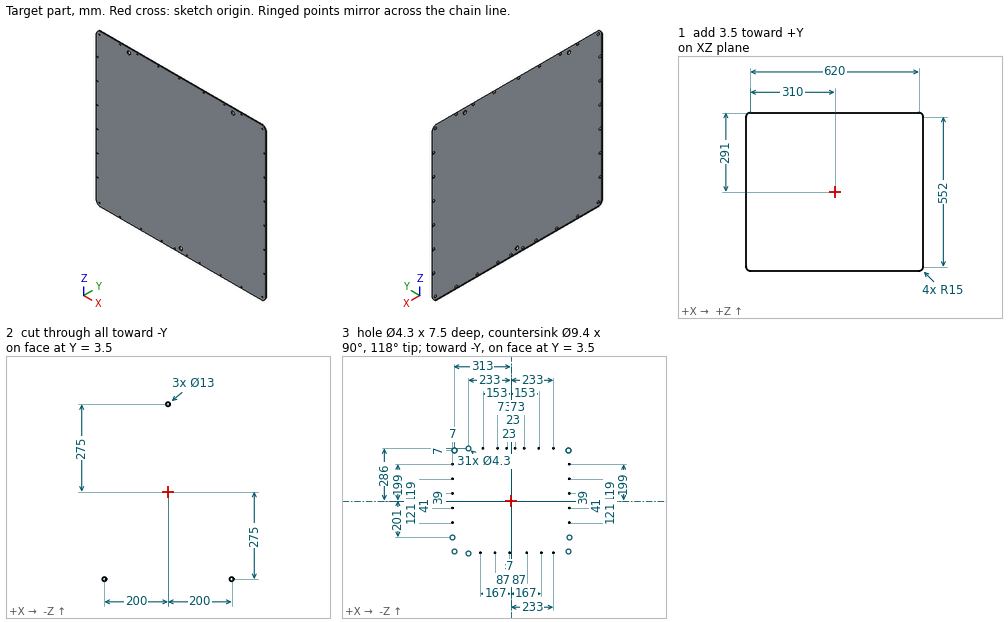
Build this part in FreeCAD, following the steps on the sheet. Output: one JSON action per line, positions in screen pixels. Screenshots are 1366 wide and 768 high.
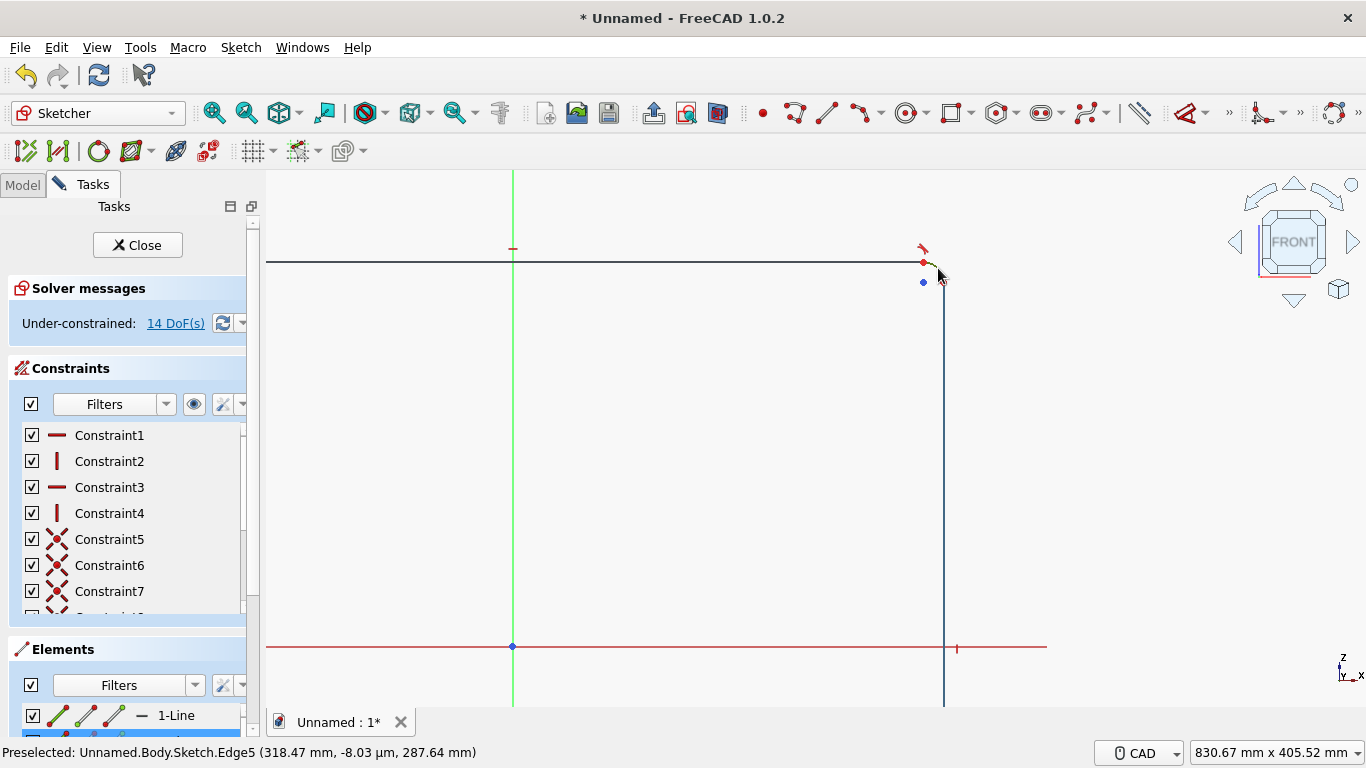
{"action": "key", "text": "t"}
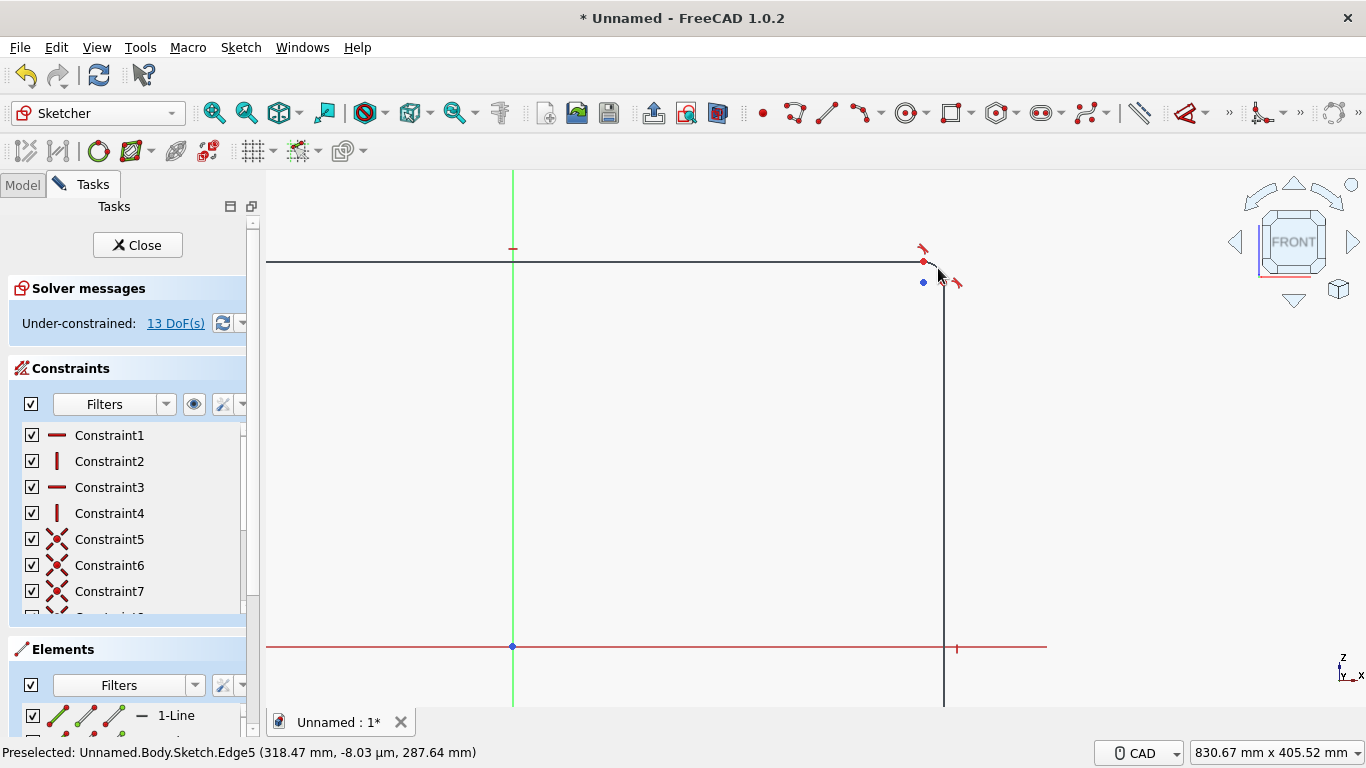
{"action": "left_click", "coordinate": [944, 502]}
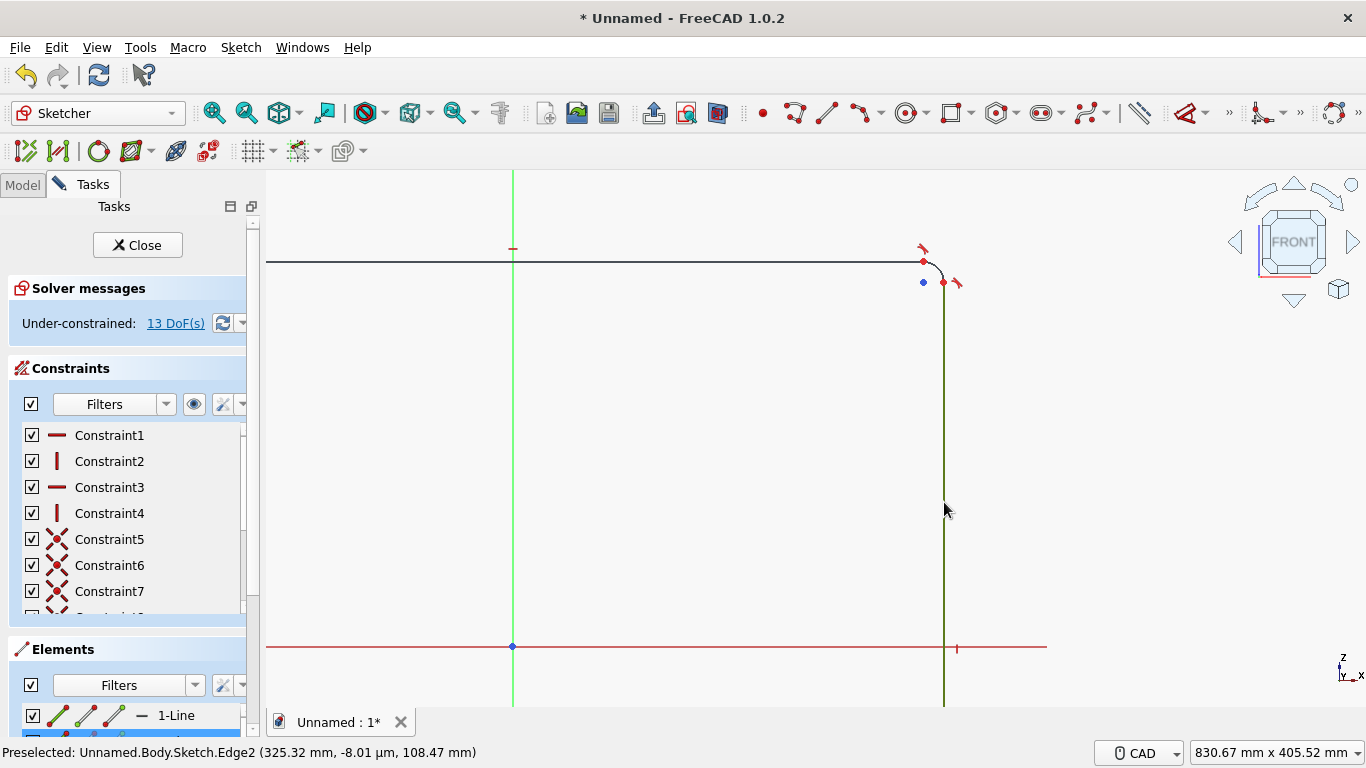
{"action": "scroll", "coordinate": [939, 269], "scroll_direction": "down", "scroll_amount": 4}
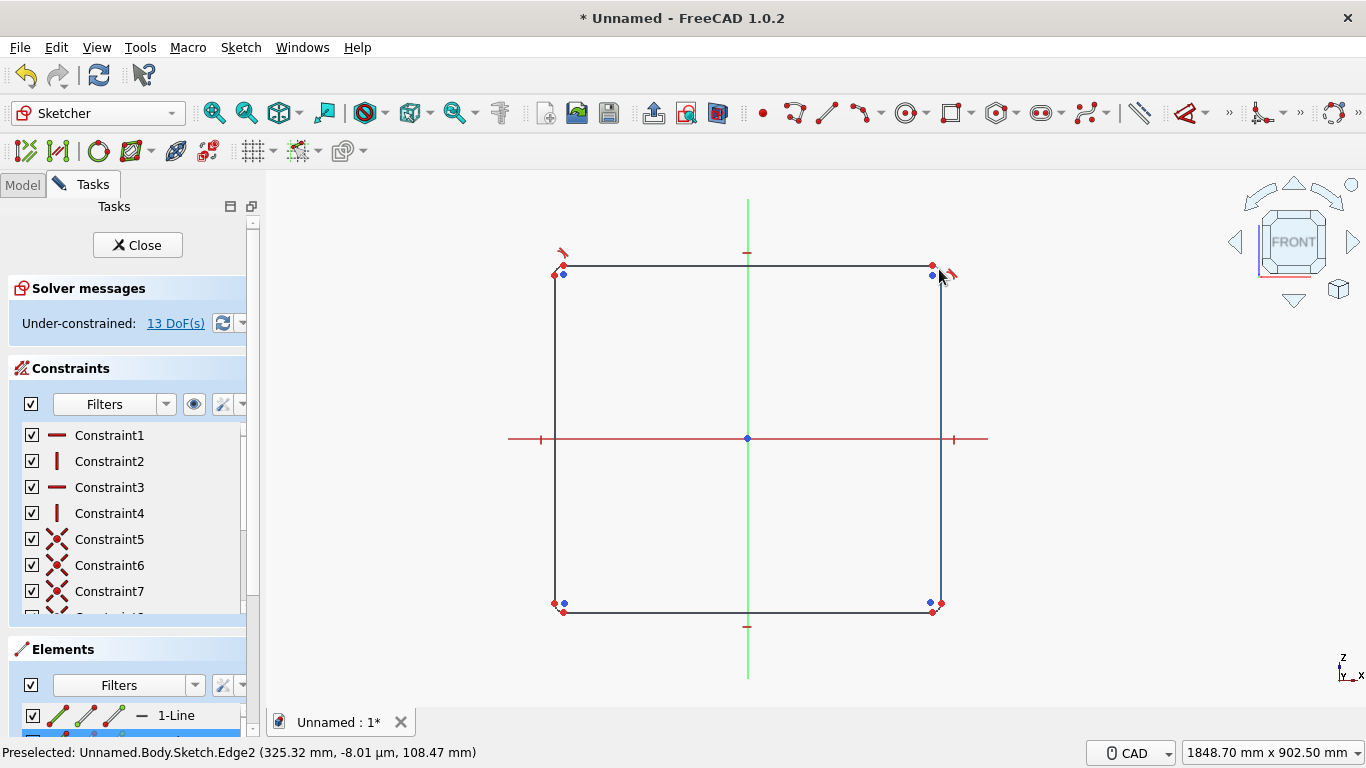
{"action": "scroll", "coordinate": [936, 611], "scroll_direction": "up", "scroll_amount": 7}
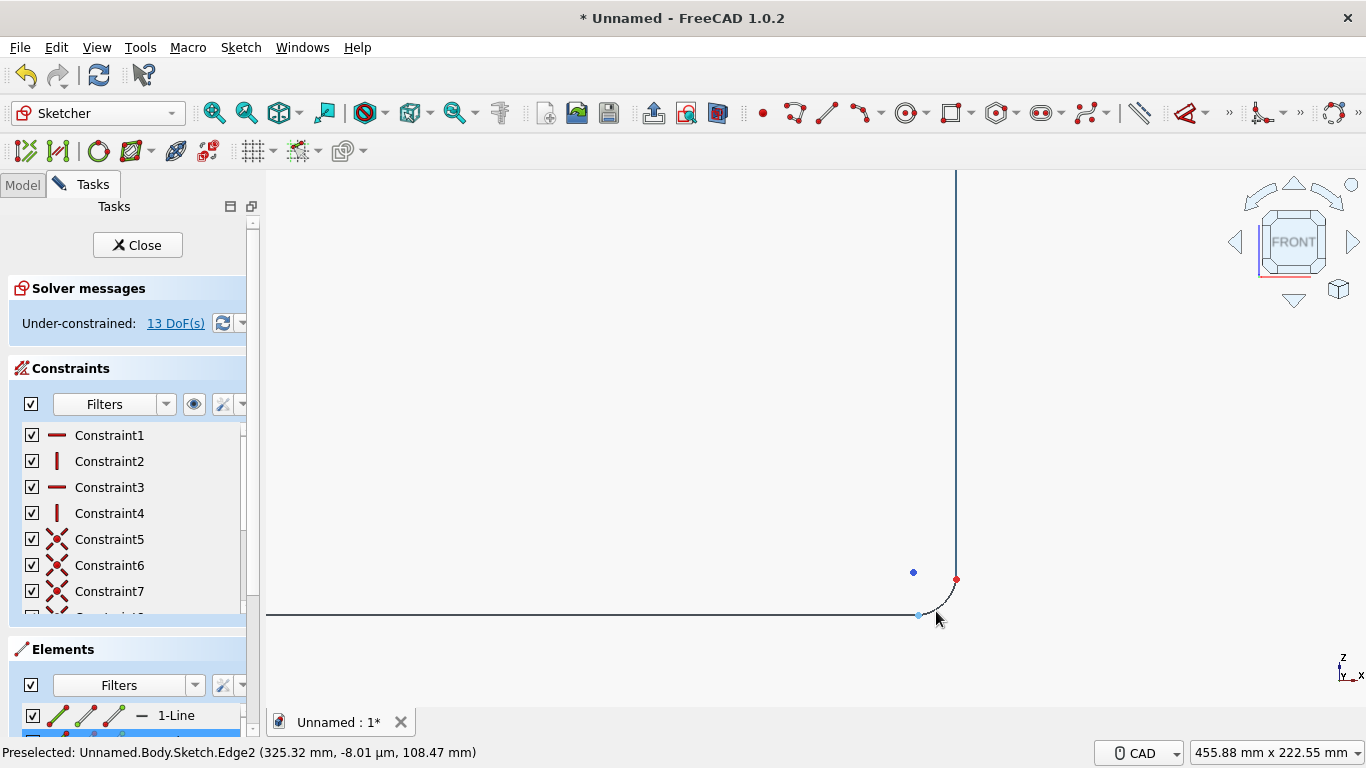
{"action": "left_click", "coordinate": [934, 610]}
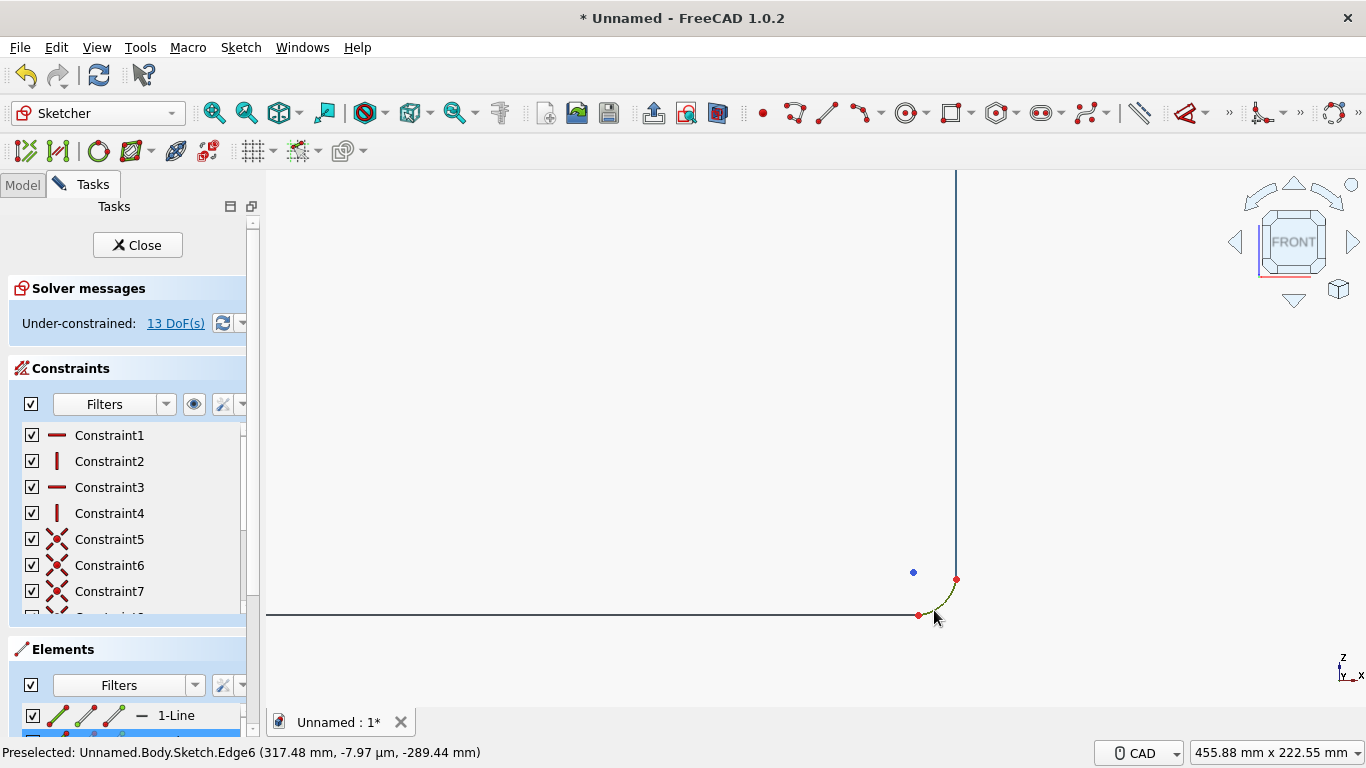
{"action": "key", "text": "t"}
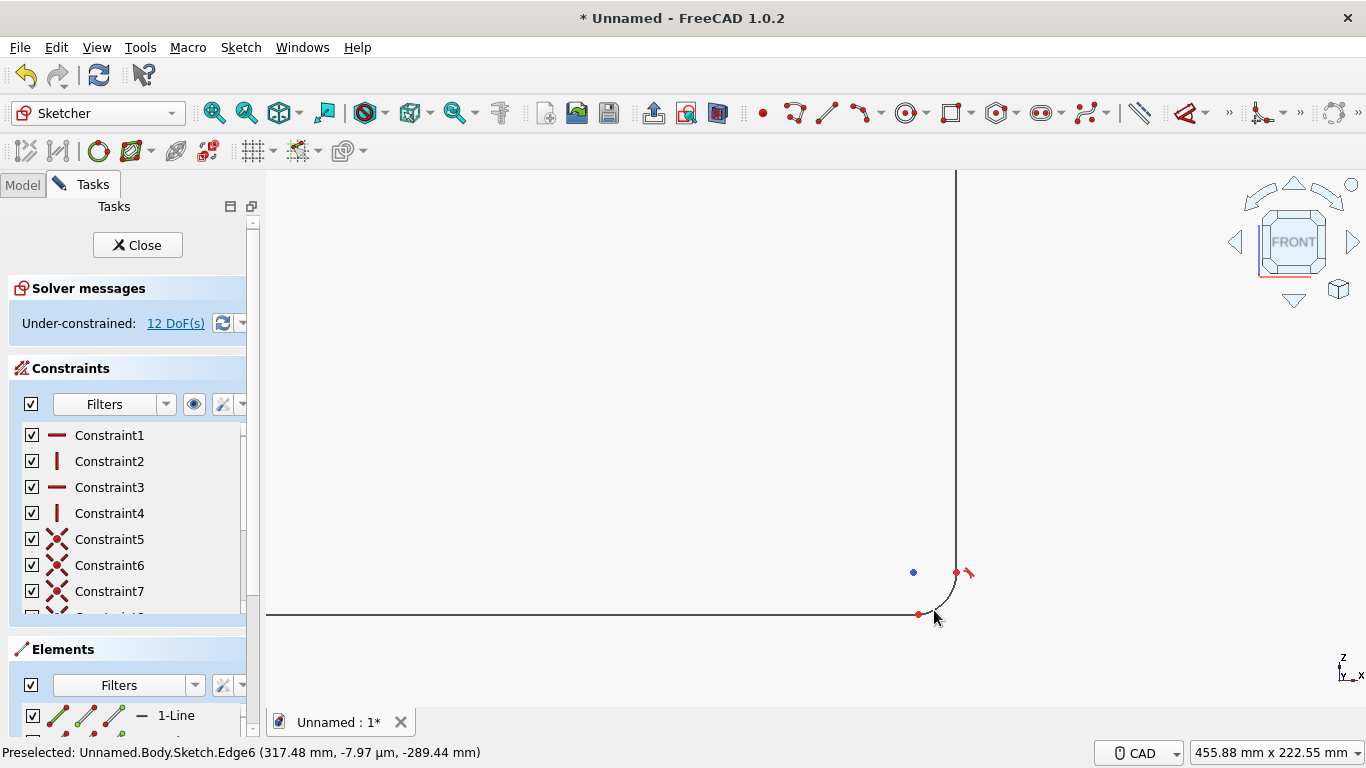
{"action": "scroll", "coordinate": [936, 611], "scroll_direction": "down", "scroll_amount": 7}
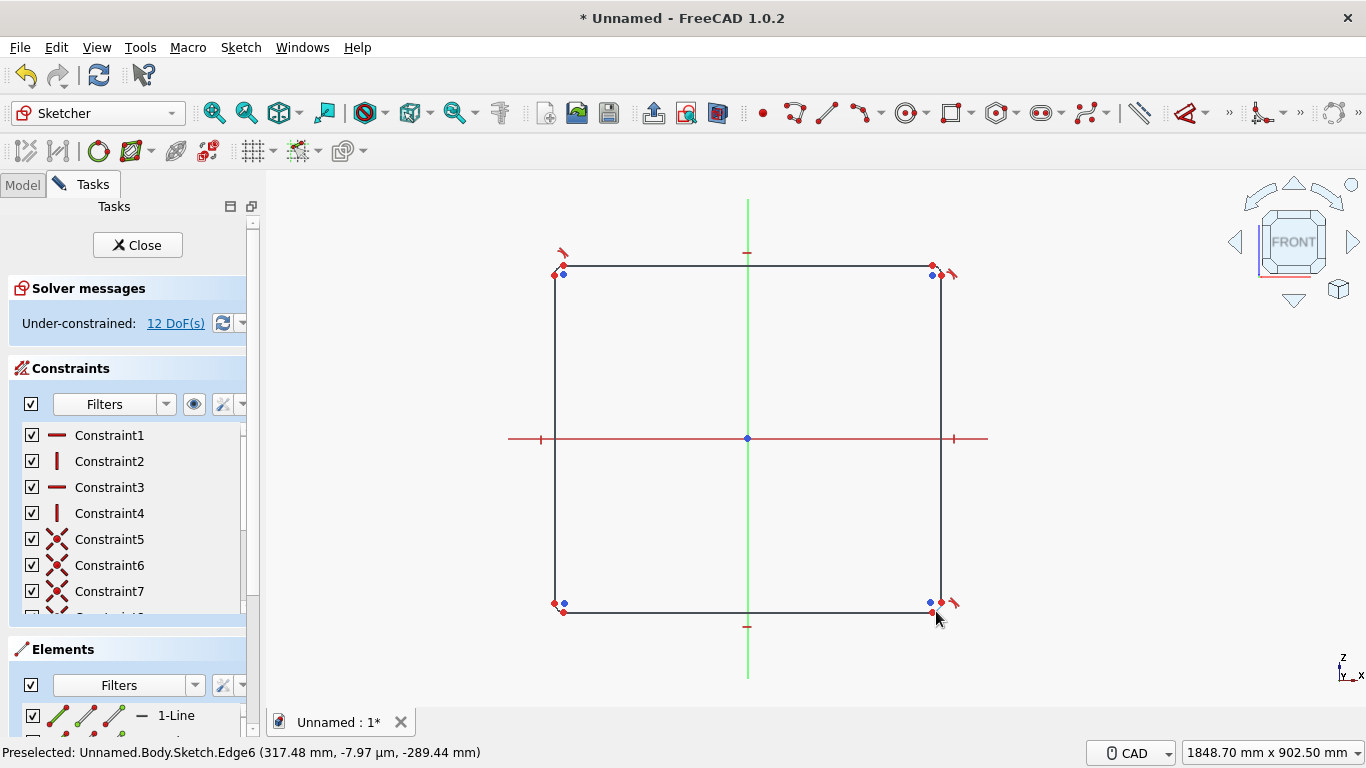
{"action": "left_click", "coordinate": [822, 613]}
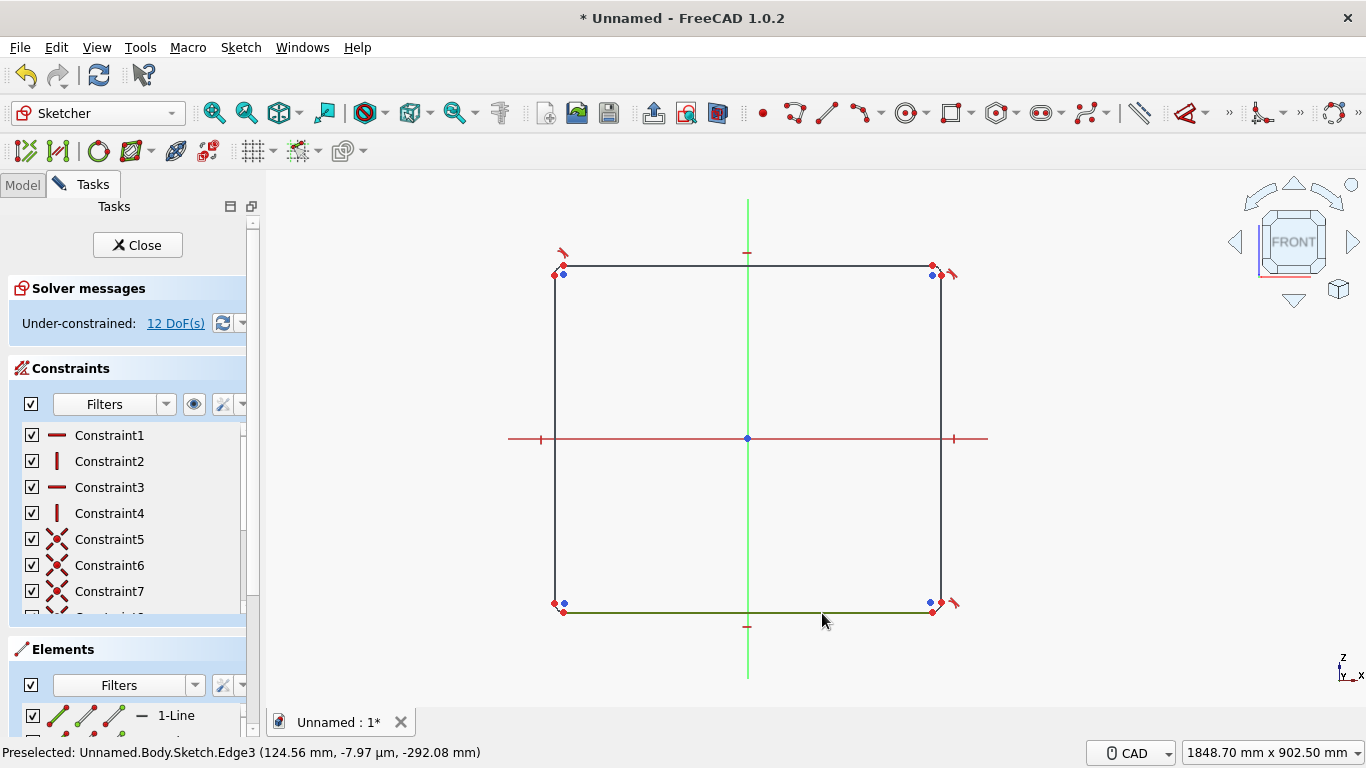
{"action": "scroll", "coordinate": [939, 609], "scroll_direction": "up", "scroll_amount": 4}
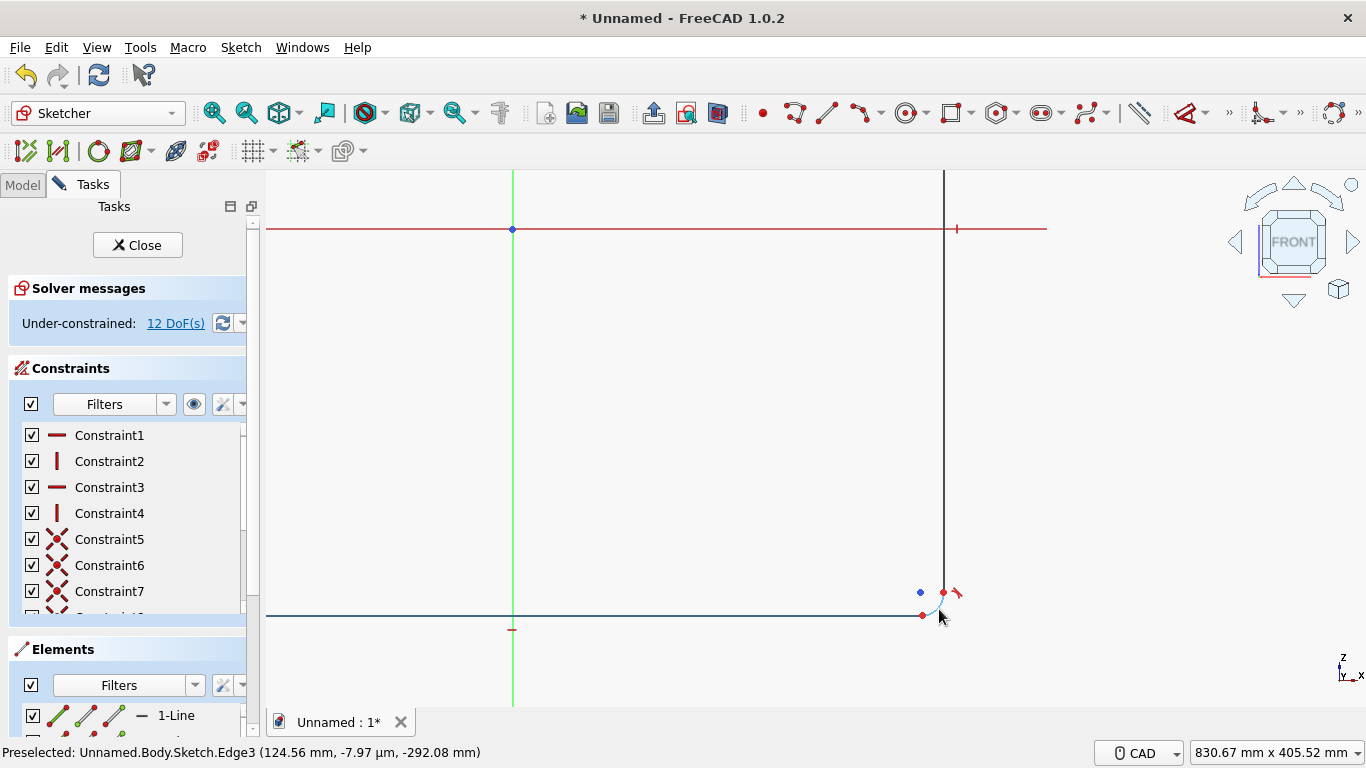
{"action": "left_click", "coordinate": [938, 608]}